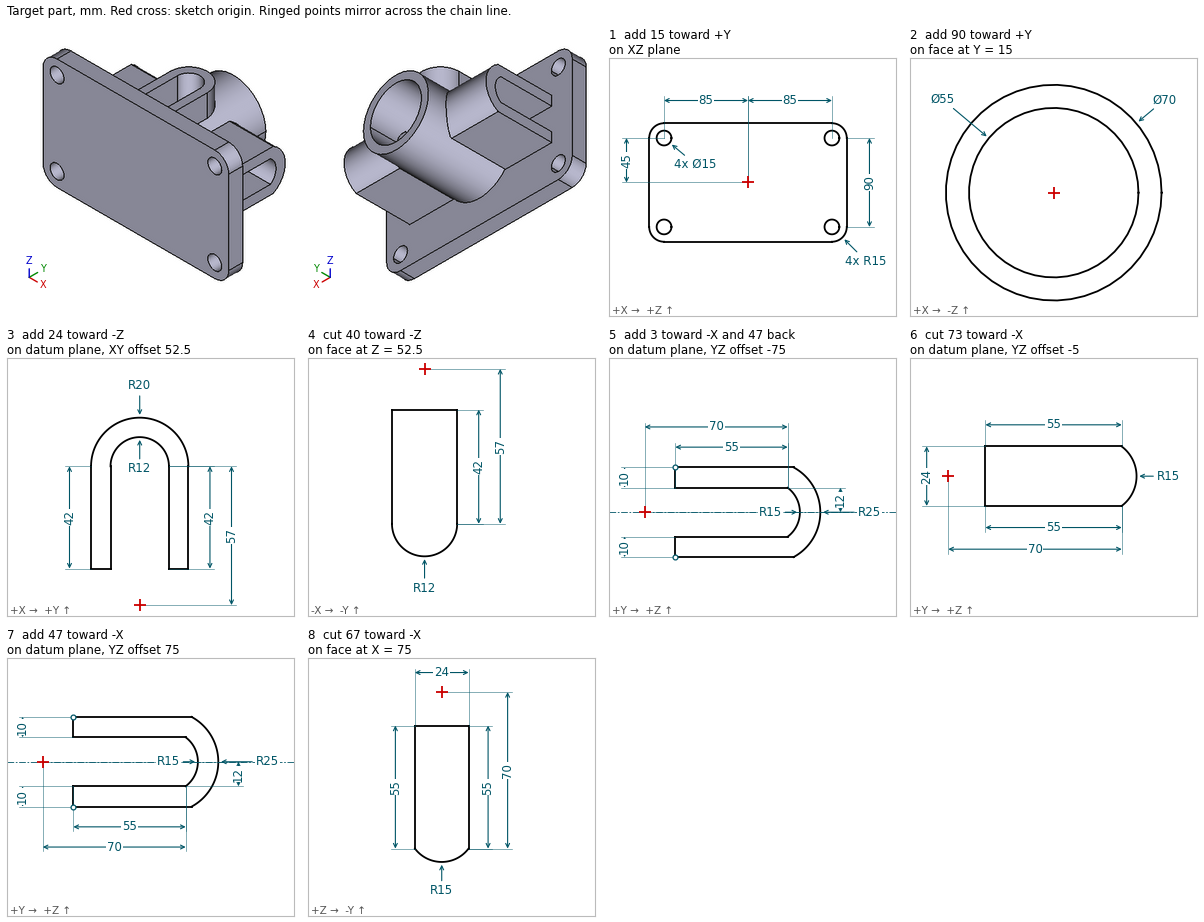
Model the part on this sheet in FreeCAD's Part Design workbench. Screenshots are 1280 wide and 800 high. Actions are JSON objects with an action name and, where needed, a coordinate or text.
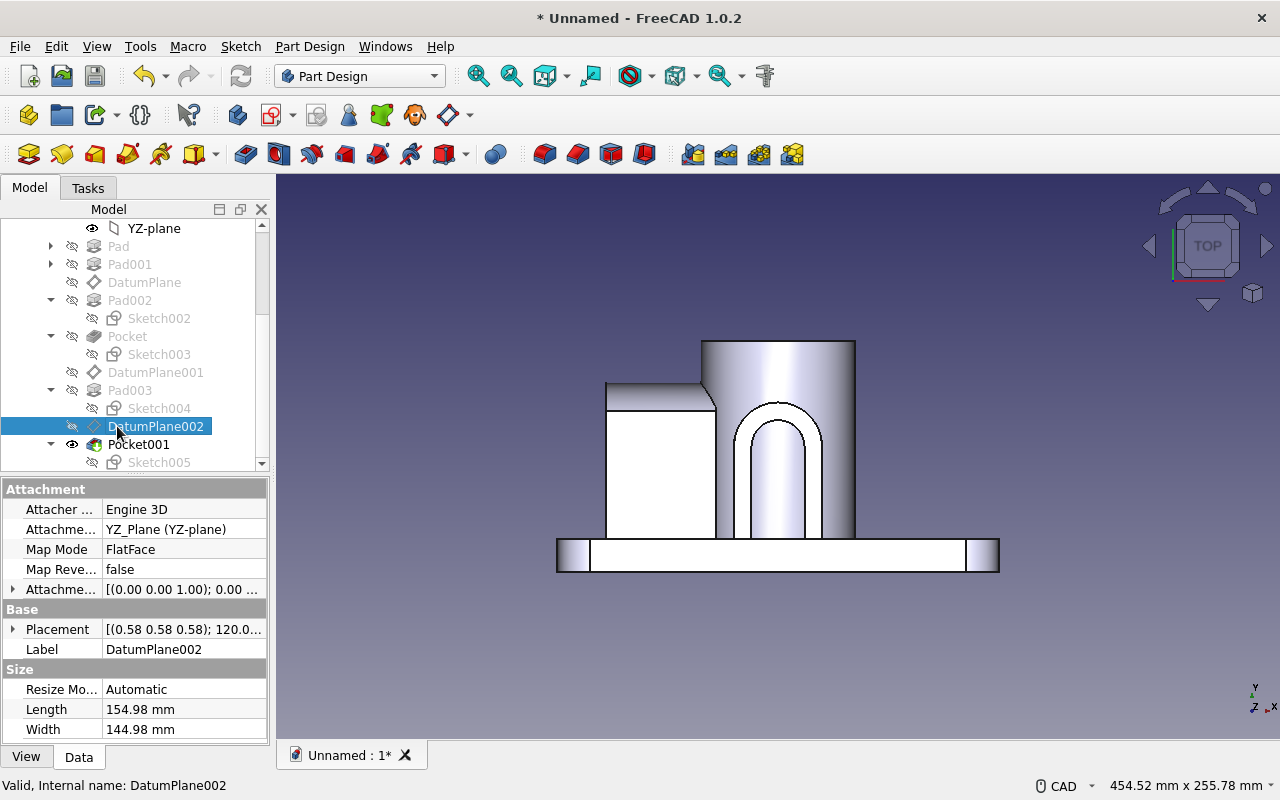
{"action": "scroll", "coordinate": [161, 350], "scroll_direction": "down", "scroll_amount": 3}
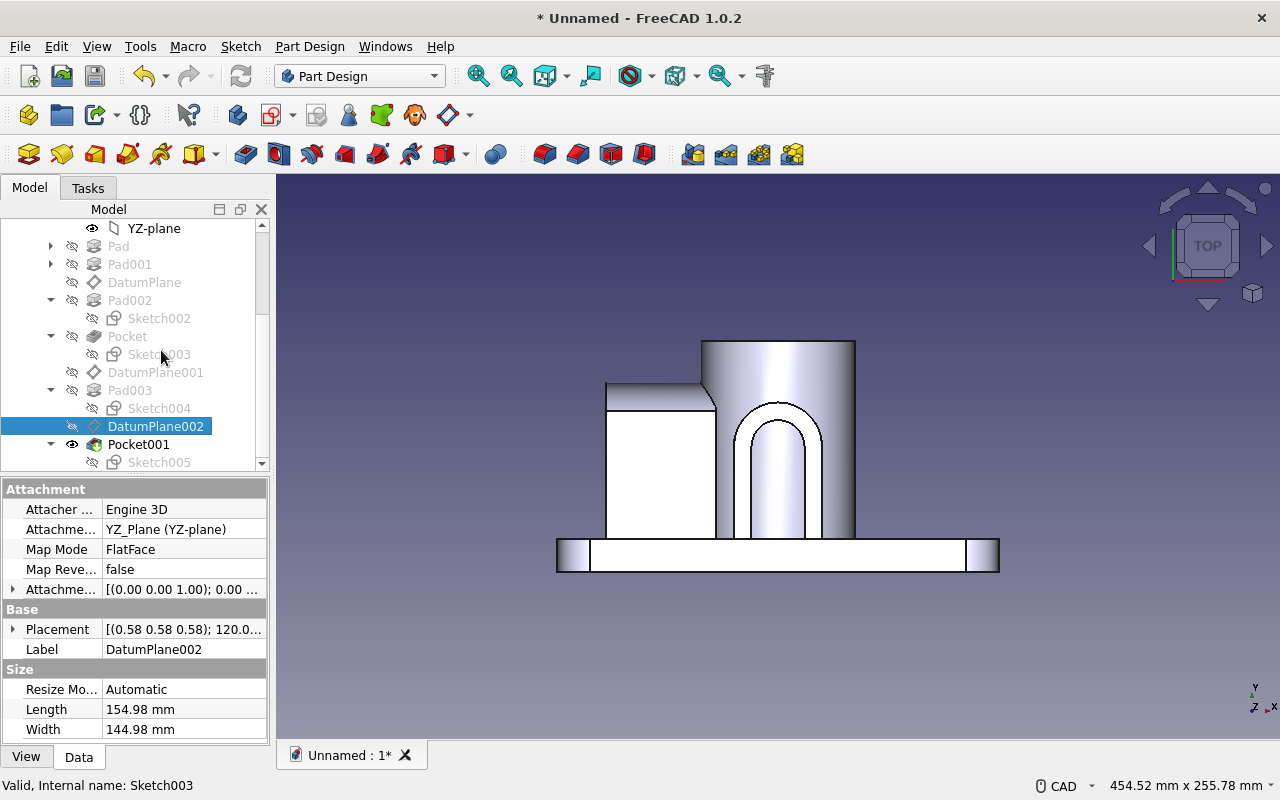
{"action": "scroll", "coordinate": [161, 350], "scroll_direction": "up", "scroll_amount": 15}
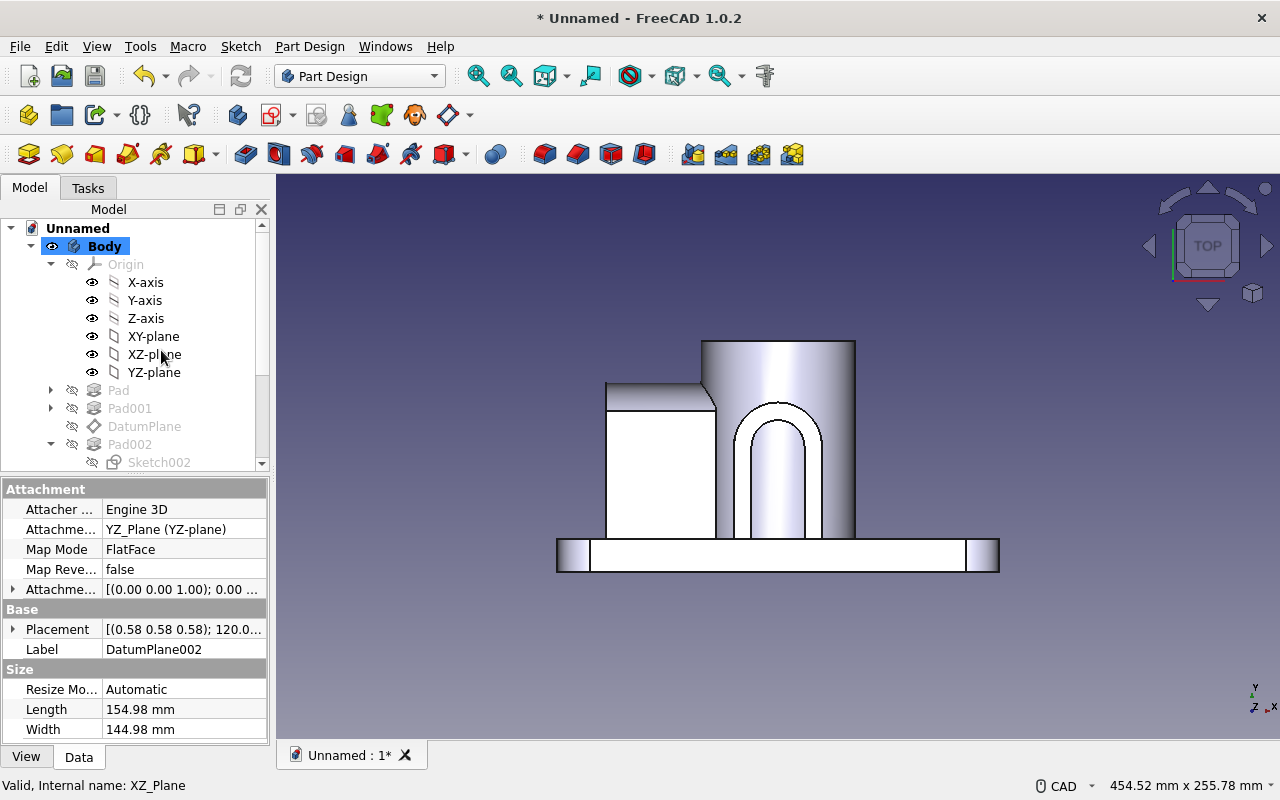
{"action": "left_click", "coordinate": [137, 372]}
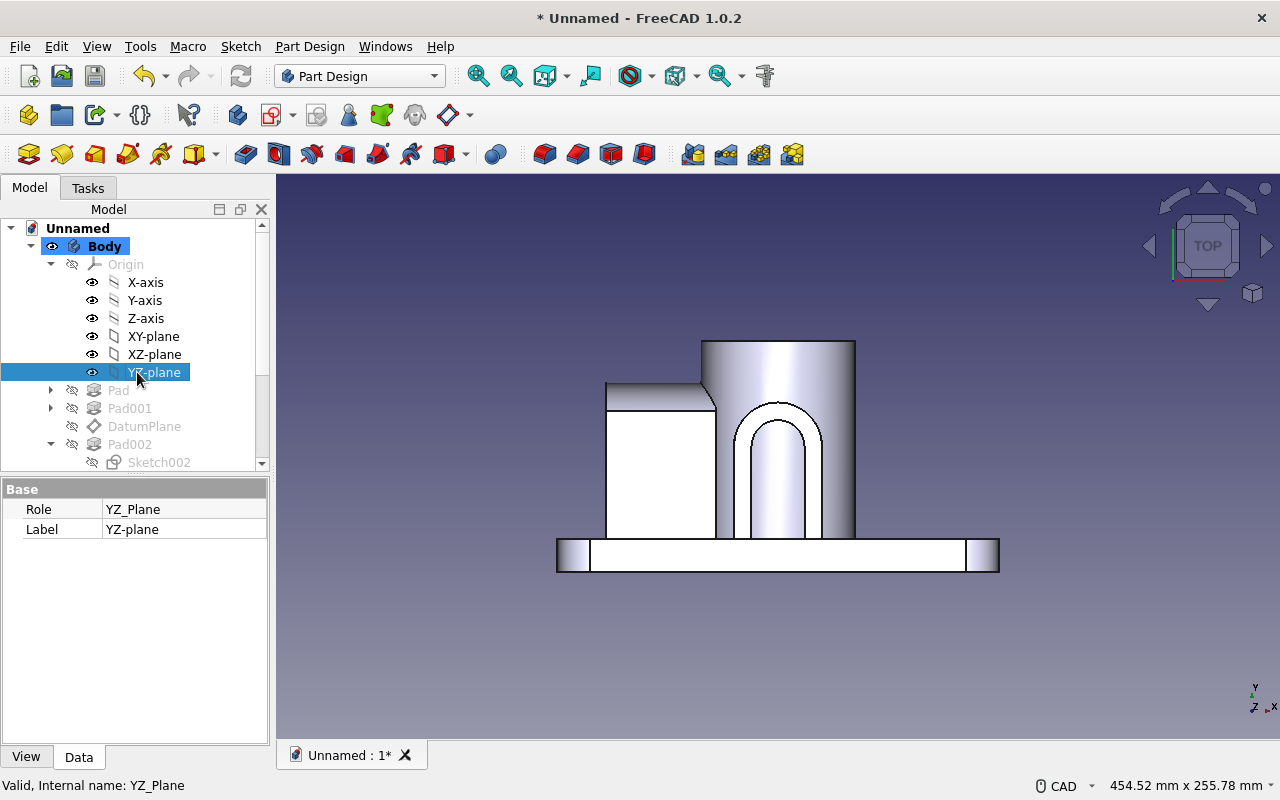
{"action": "left_click", "coordinate": [448, 116]}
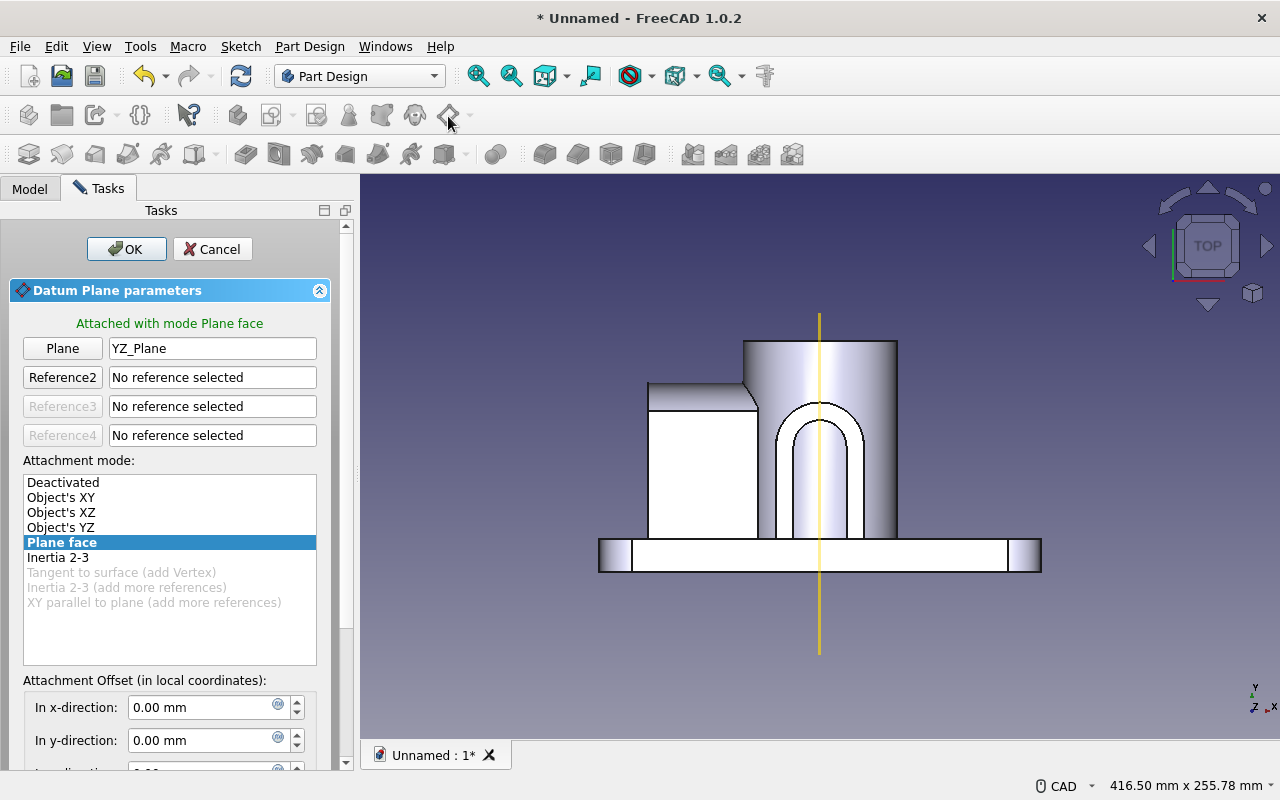
{"action": "scroll", "coordinate": [346, 495], "scroll_direction": "down", "scroll_amount": 2}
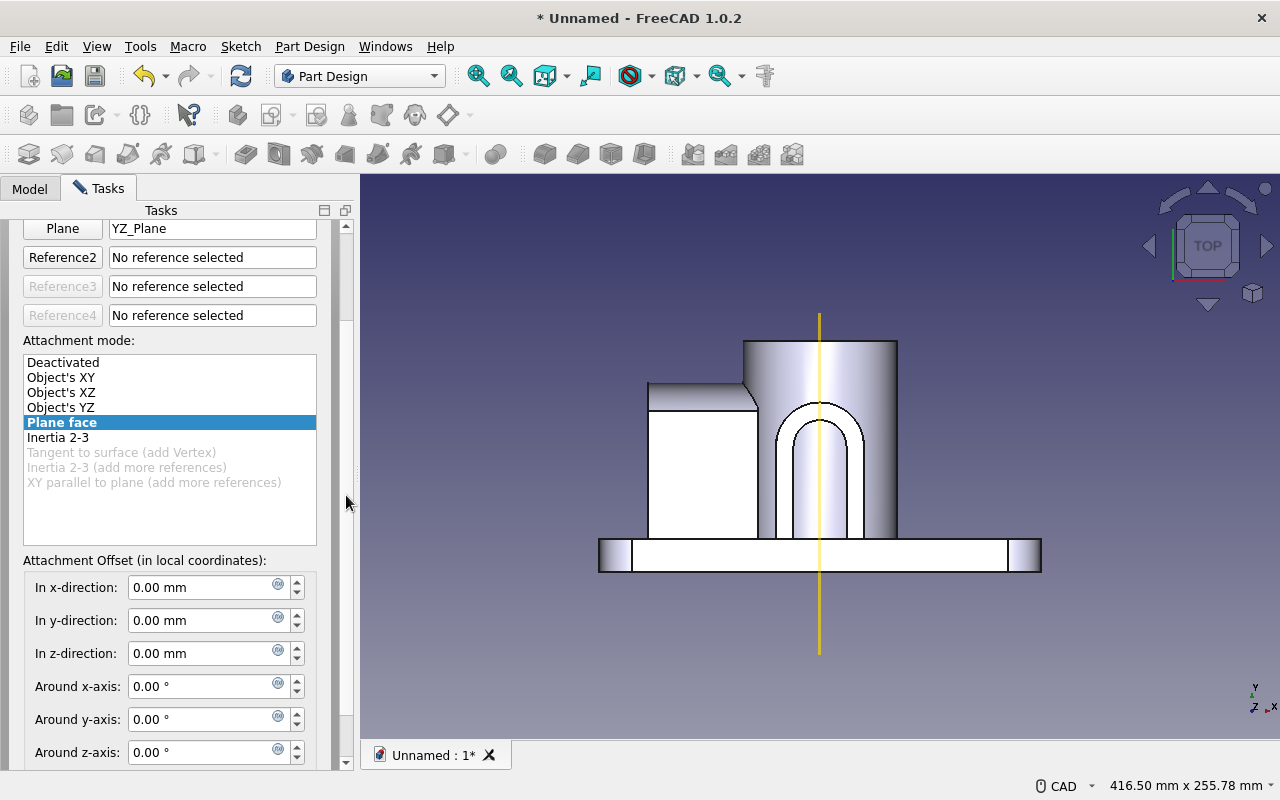
{"action": "triple_click", "coordinate": [210, 654]}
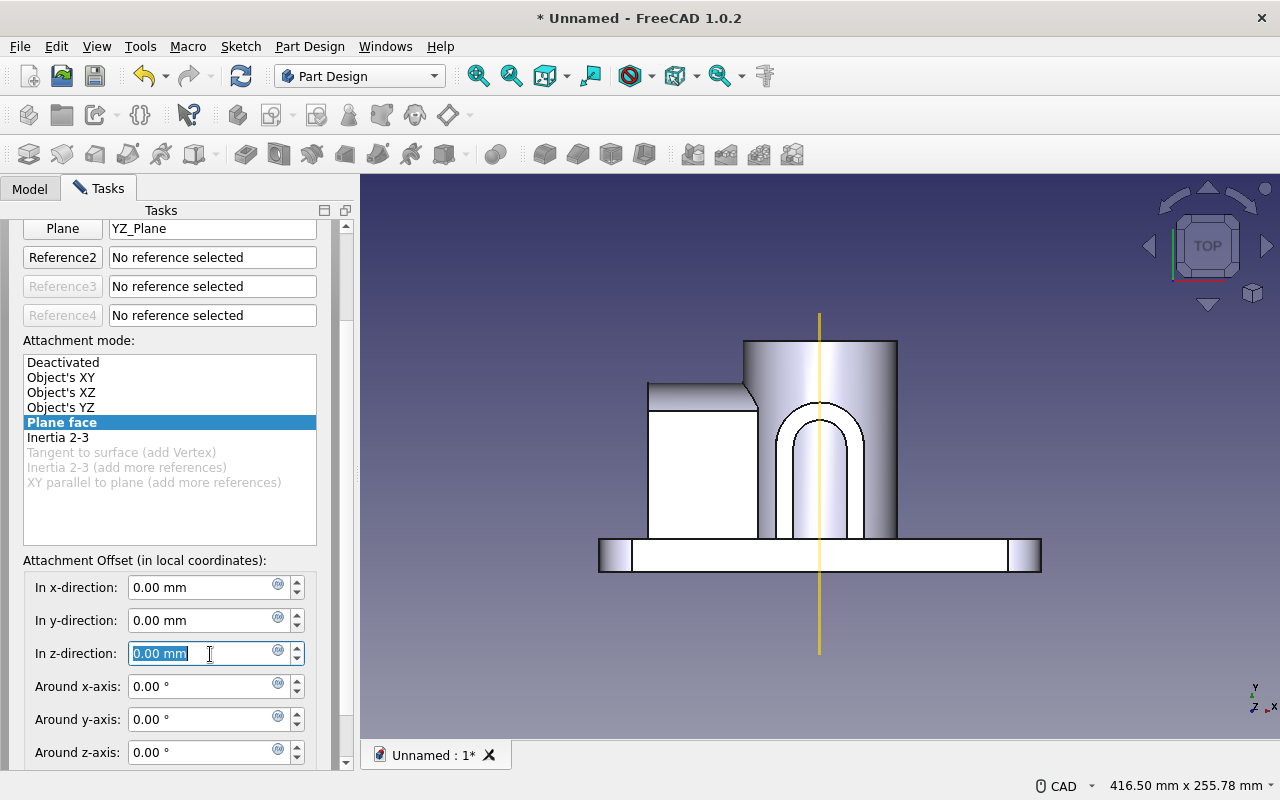
{"action": "type", "text": "75"}
{"action": "key", "text": "Tab"}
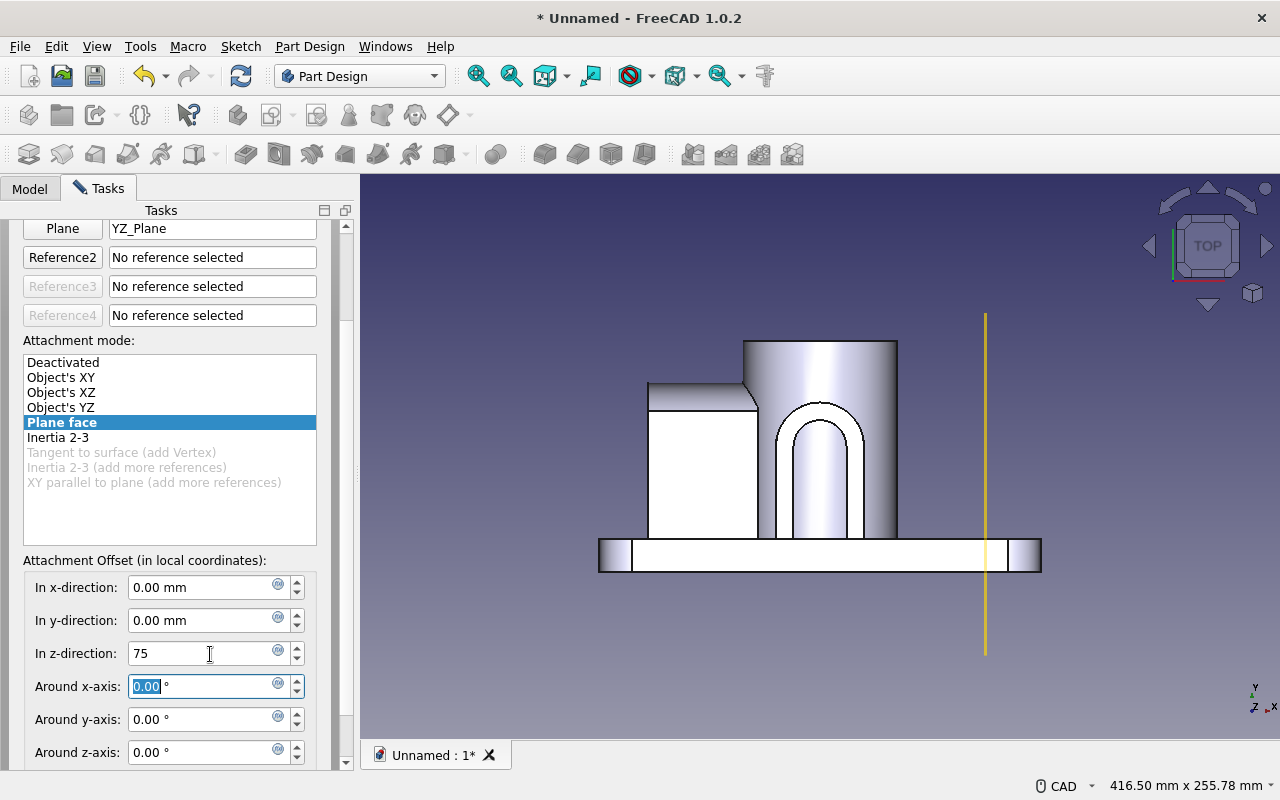
{"action": "scroll", "coordinate": [346, 495], "scroll_direction": "up", "scroll_amount": 3}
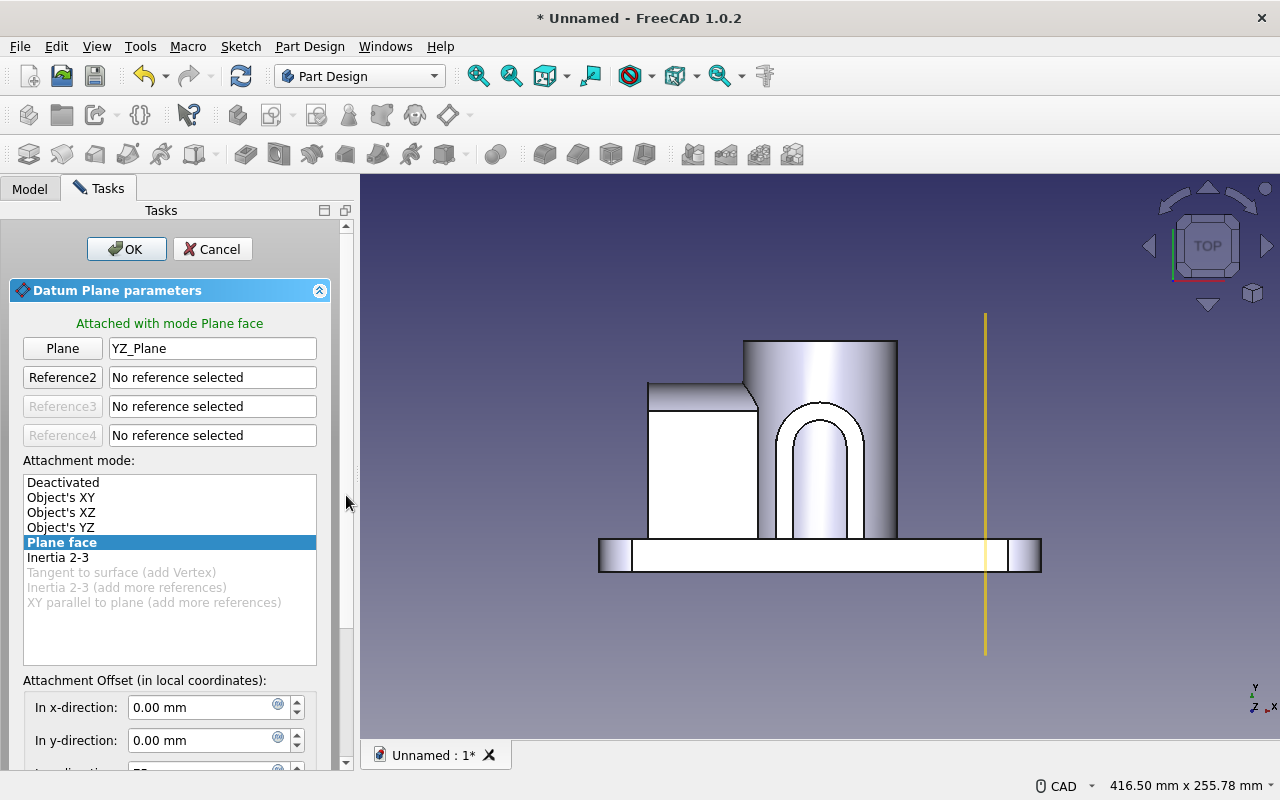
{"action": "left_click", "coordinate": [127, 249]}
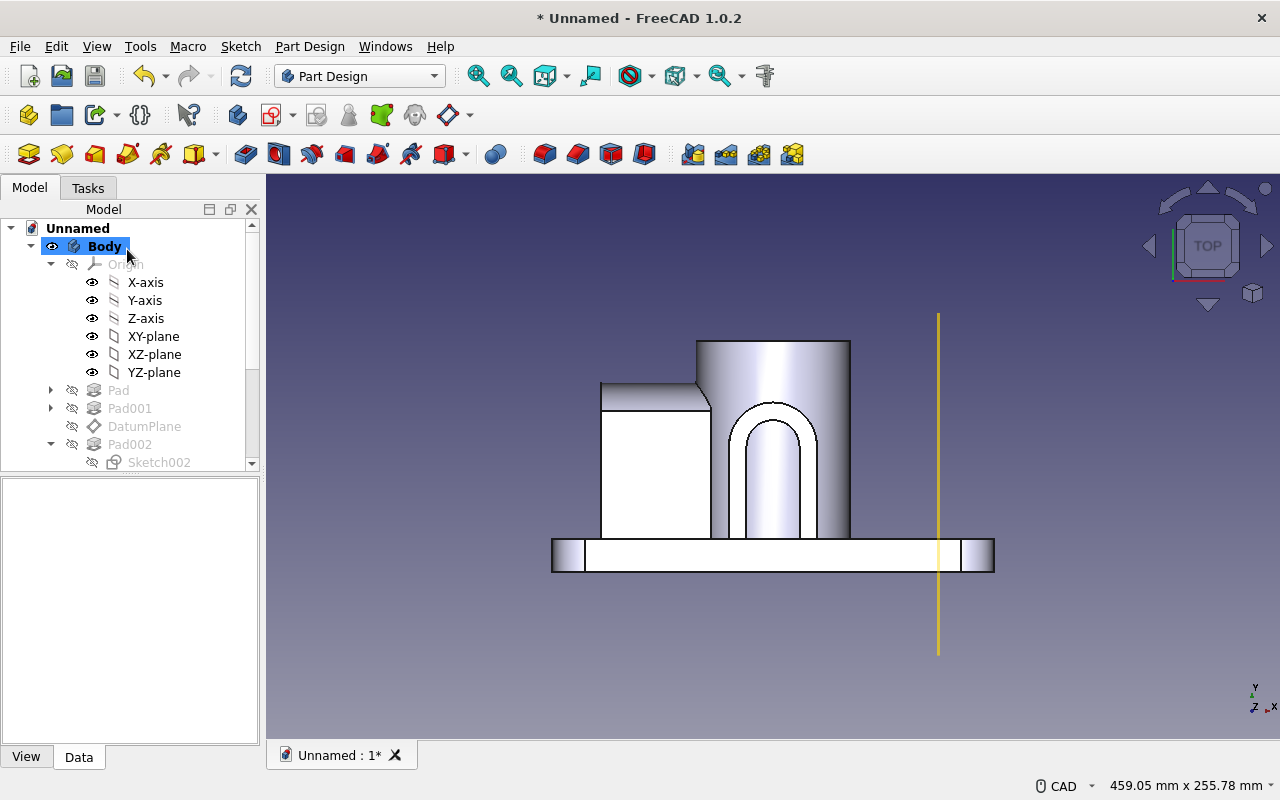
{"action": "scroll", "coordinate": [101, 350], "scroll_direction": "down", "scroll_amount": 3}